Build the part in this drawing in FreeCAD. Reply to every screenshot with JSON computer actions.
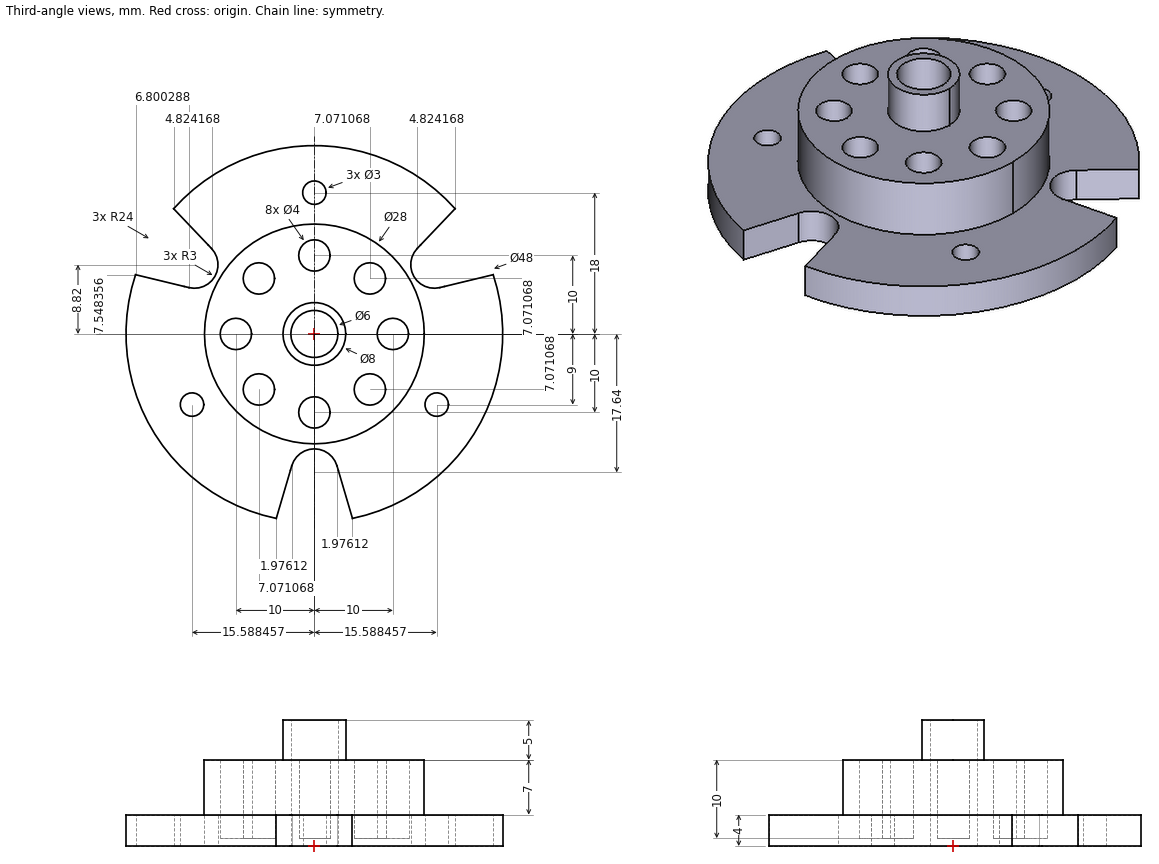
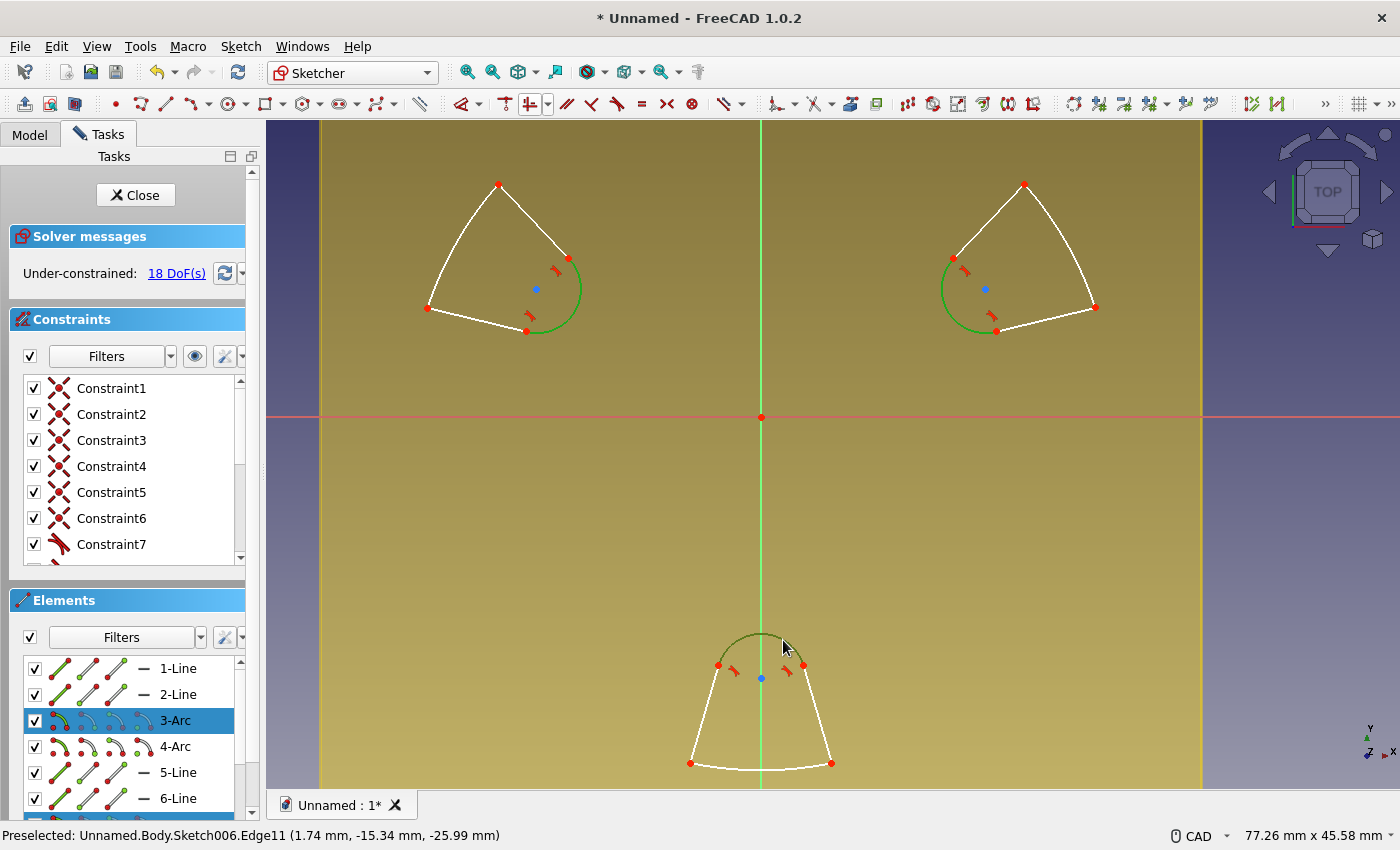
{"action": "key", "text": "e"}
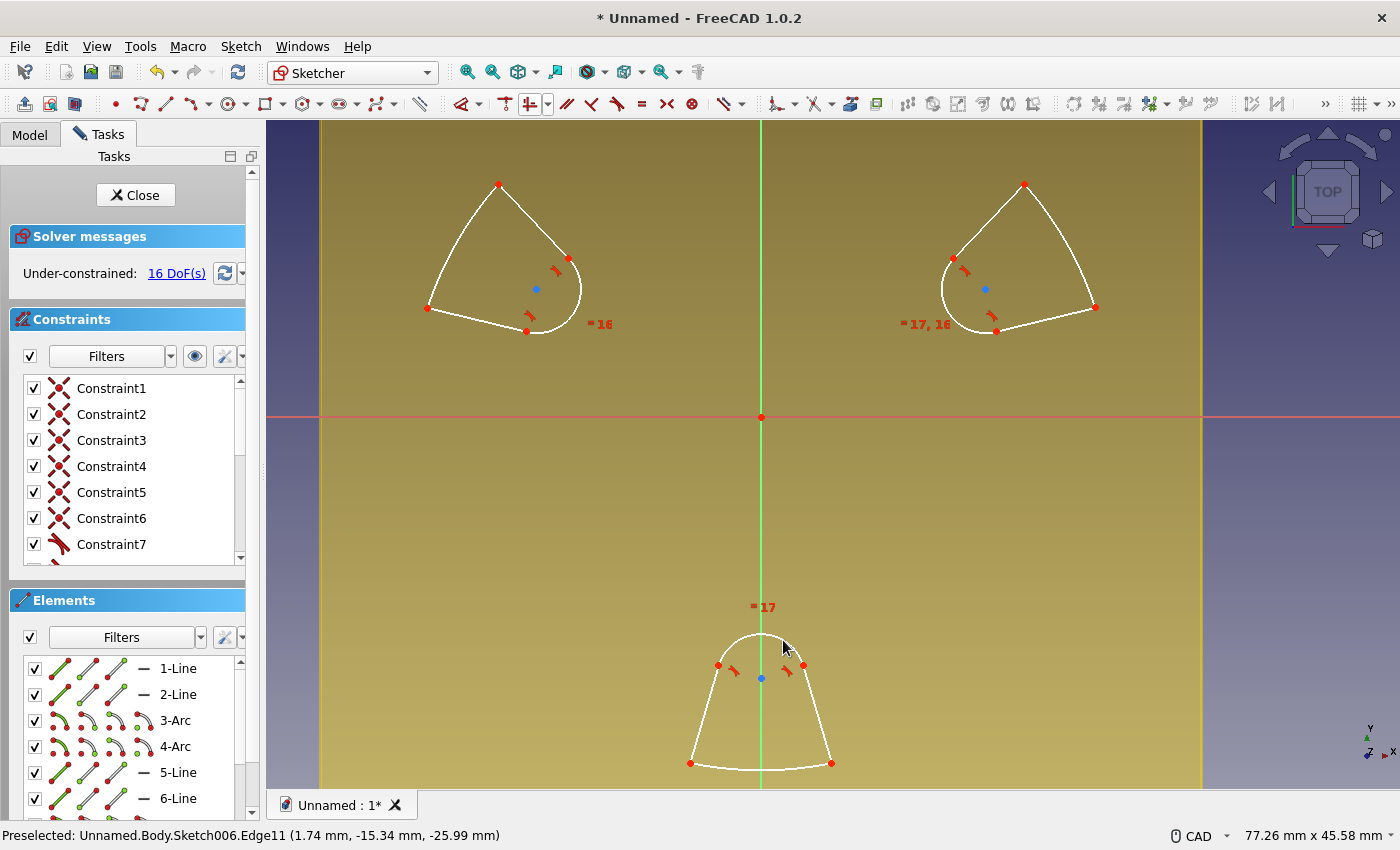
{"action": "left_click", "coordinate": [472, 218]}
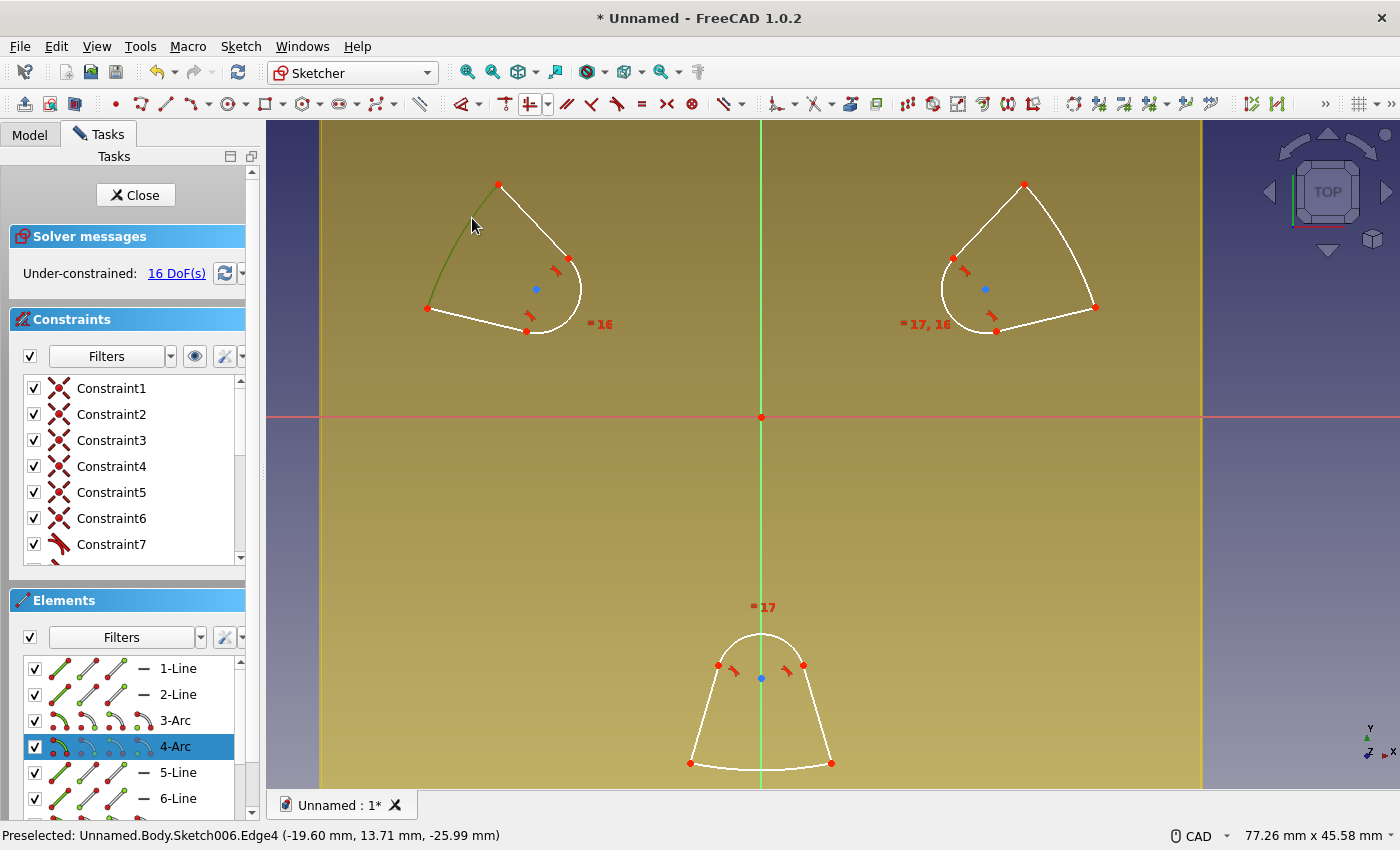
{"action": "left_click", "coordinate": [1079, 268]}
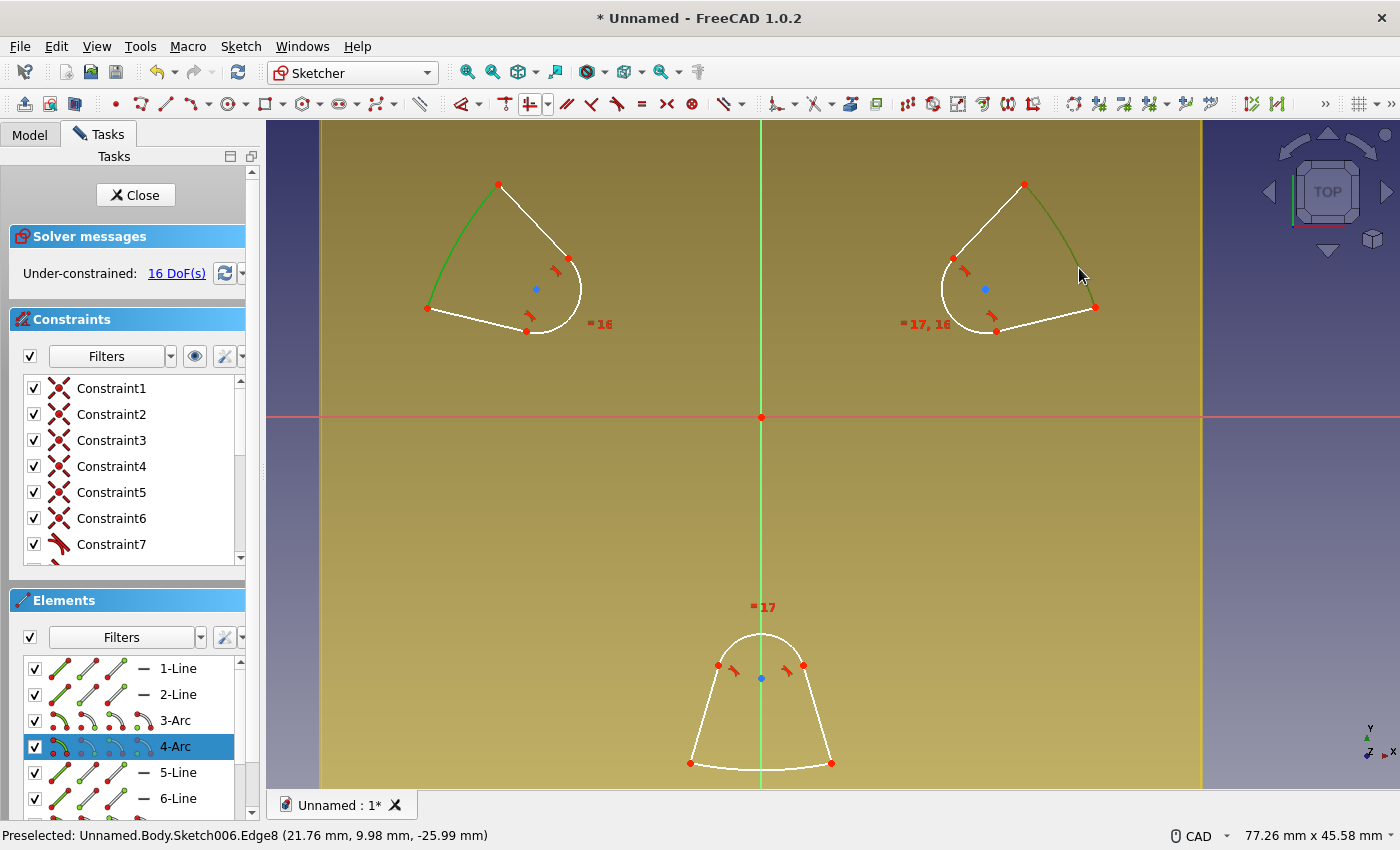
{"action": "scroll", "coordinate": [771, 411], "scroll_direction": "down", "scroll_amount": 2}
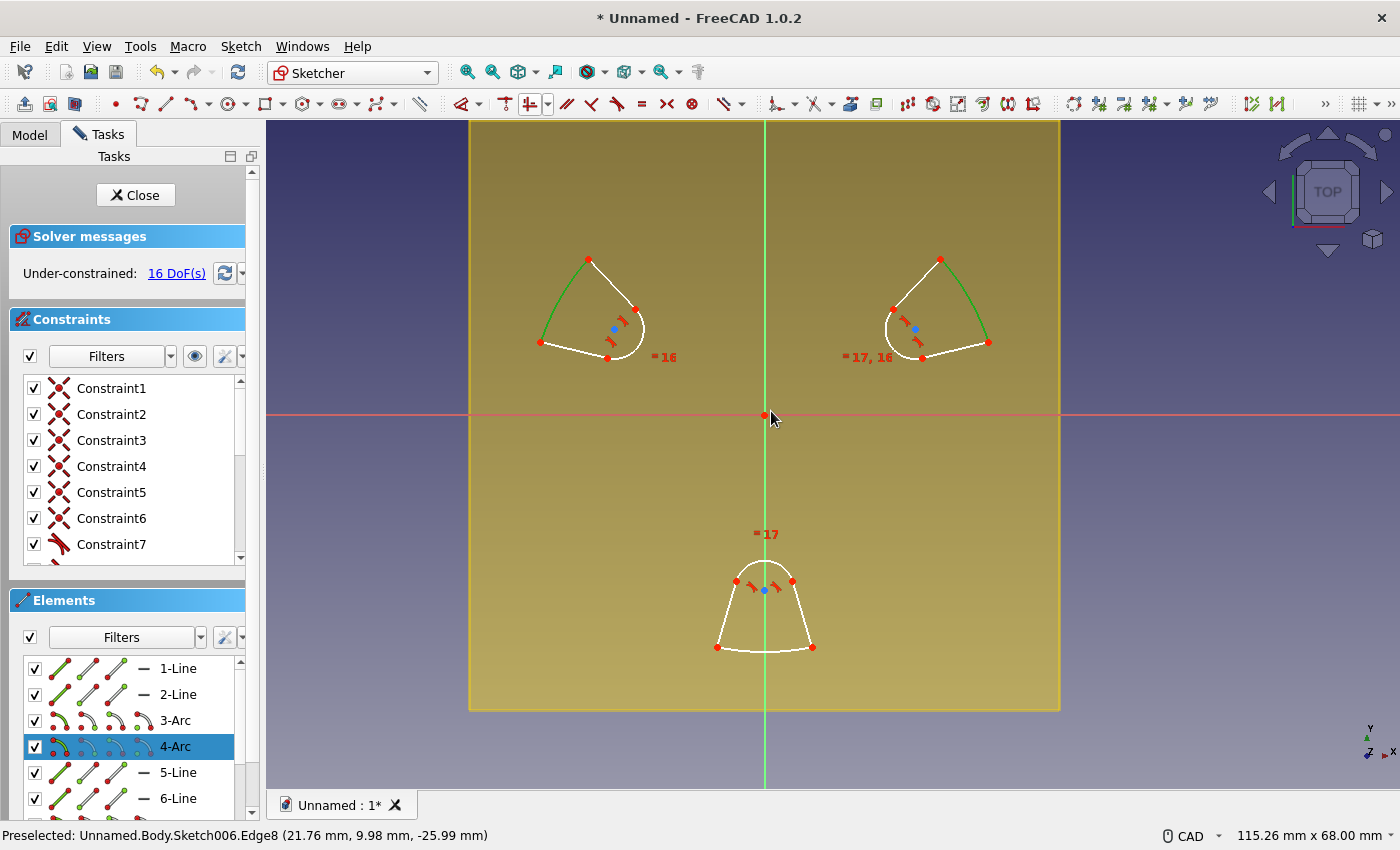
{"action": "left_click", "coordinate": [745, 651]}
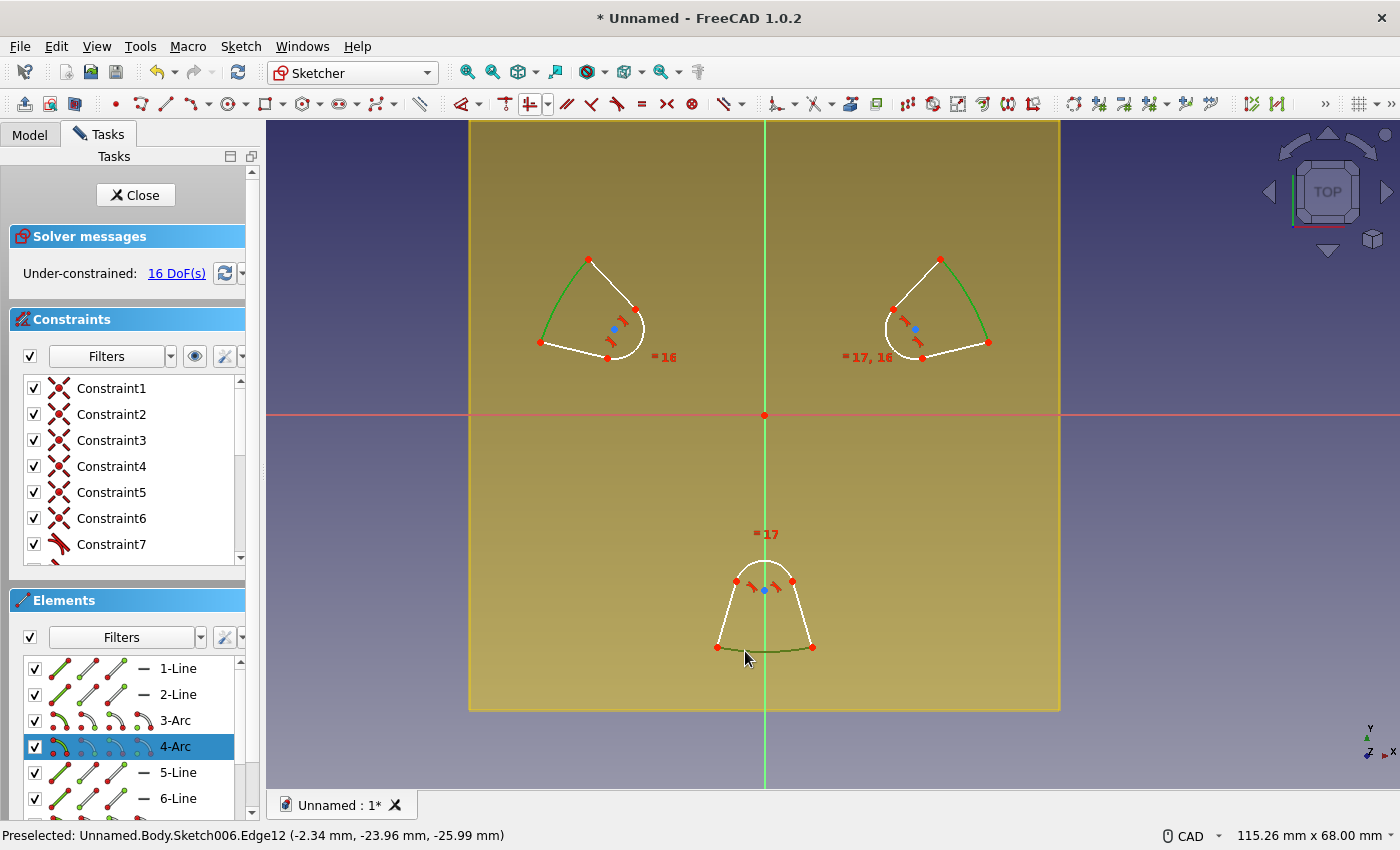
{"action": "left_click", "coordinate": [642, 104]}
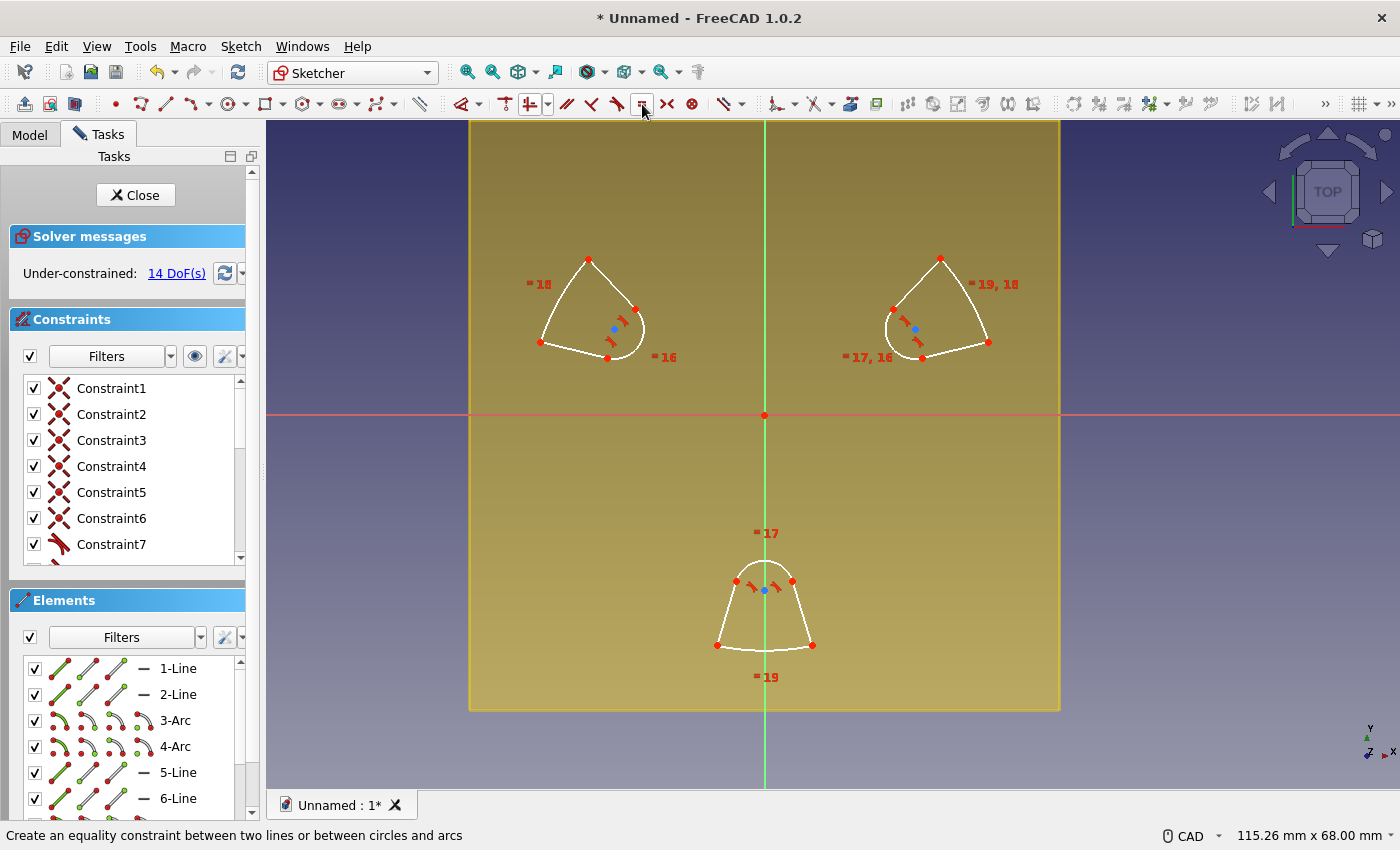
{"action": "left_click", "coordinate": [764, 590]}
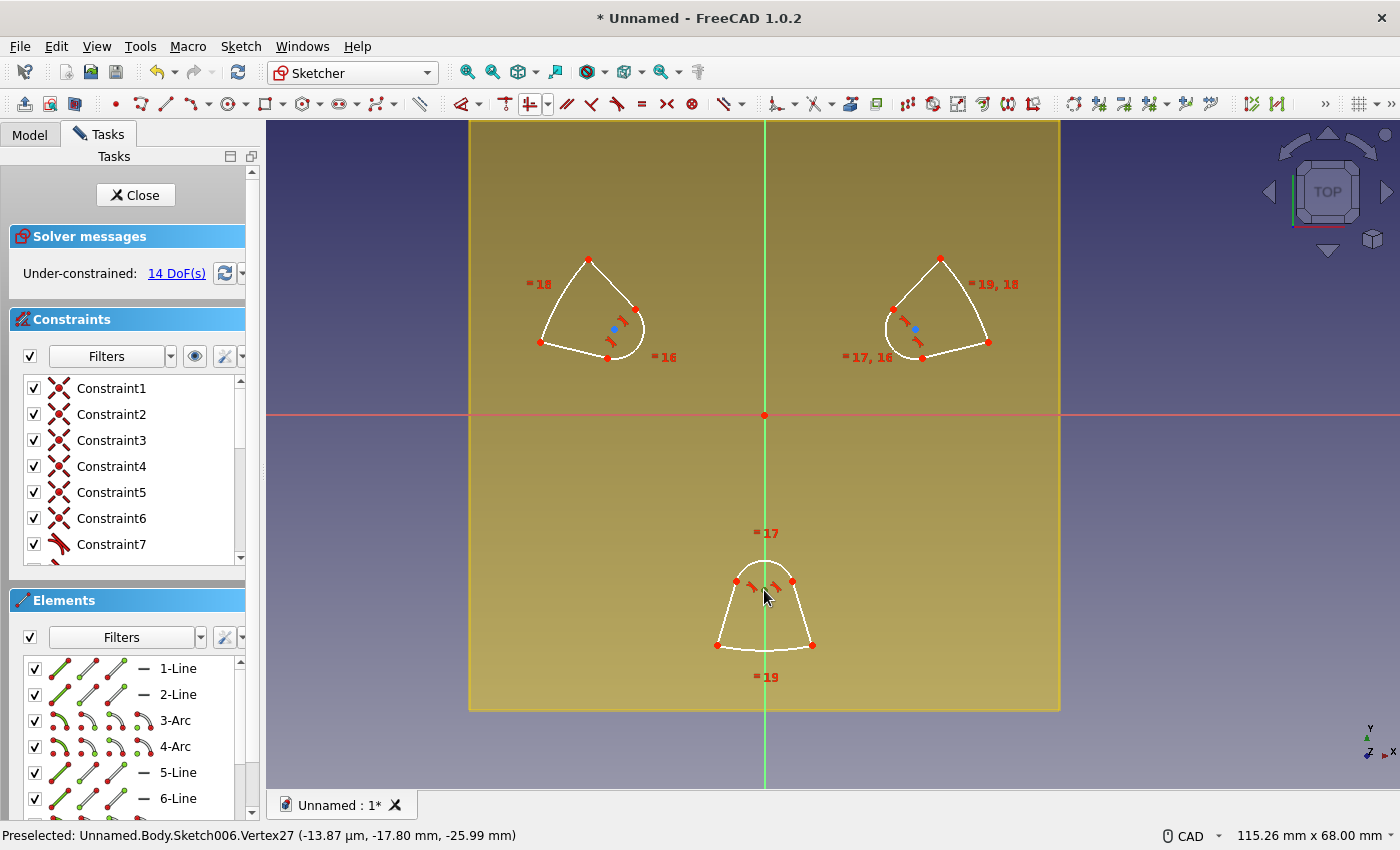
{"action": "left_click", "coordinate": [765, 717]}